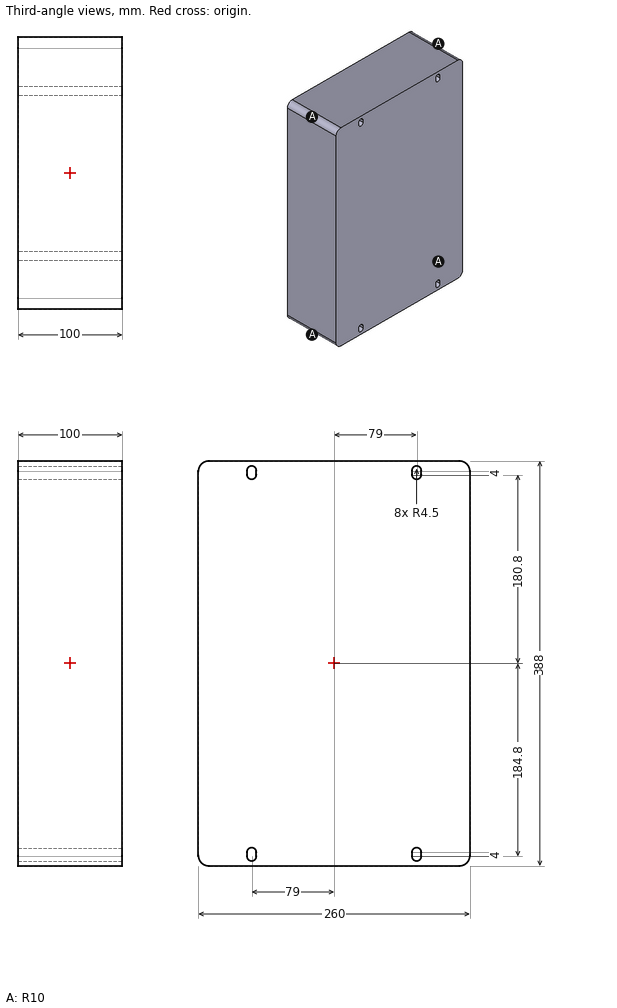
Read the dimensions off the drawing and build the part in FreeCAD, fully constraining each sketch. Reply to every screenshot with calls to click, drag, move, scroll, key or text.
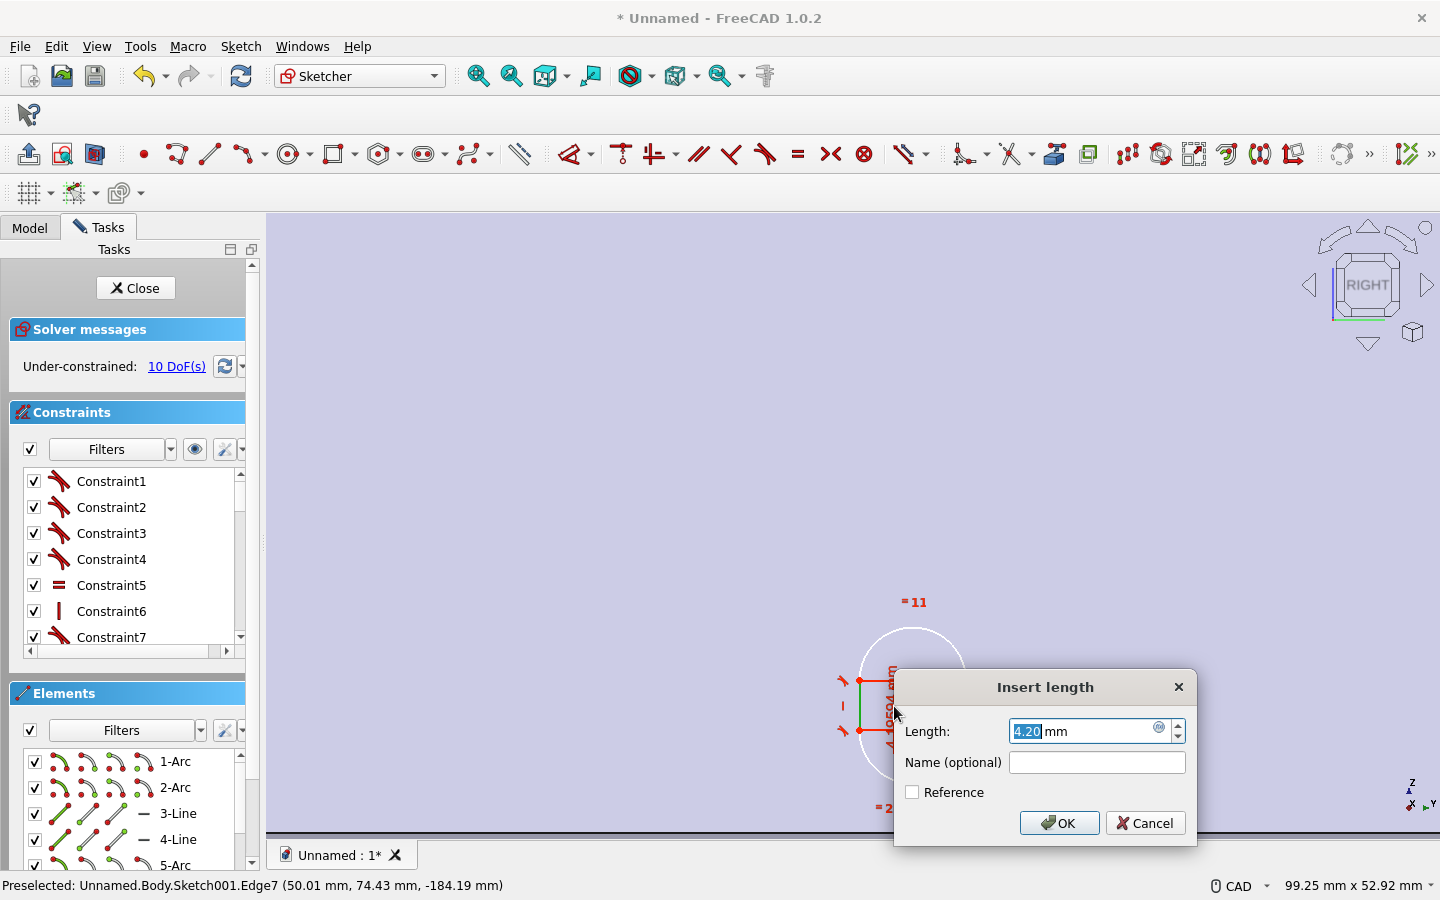
text(4)
key(Return)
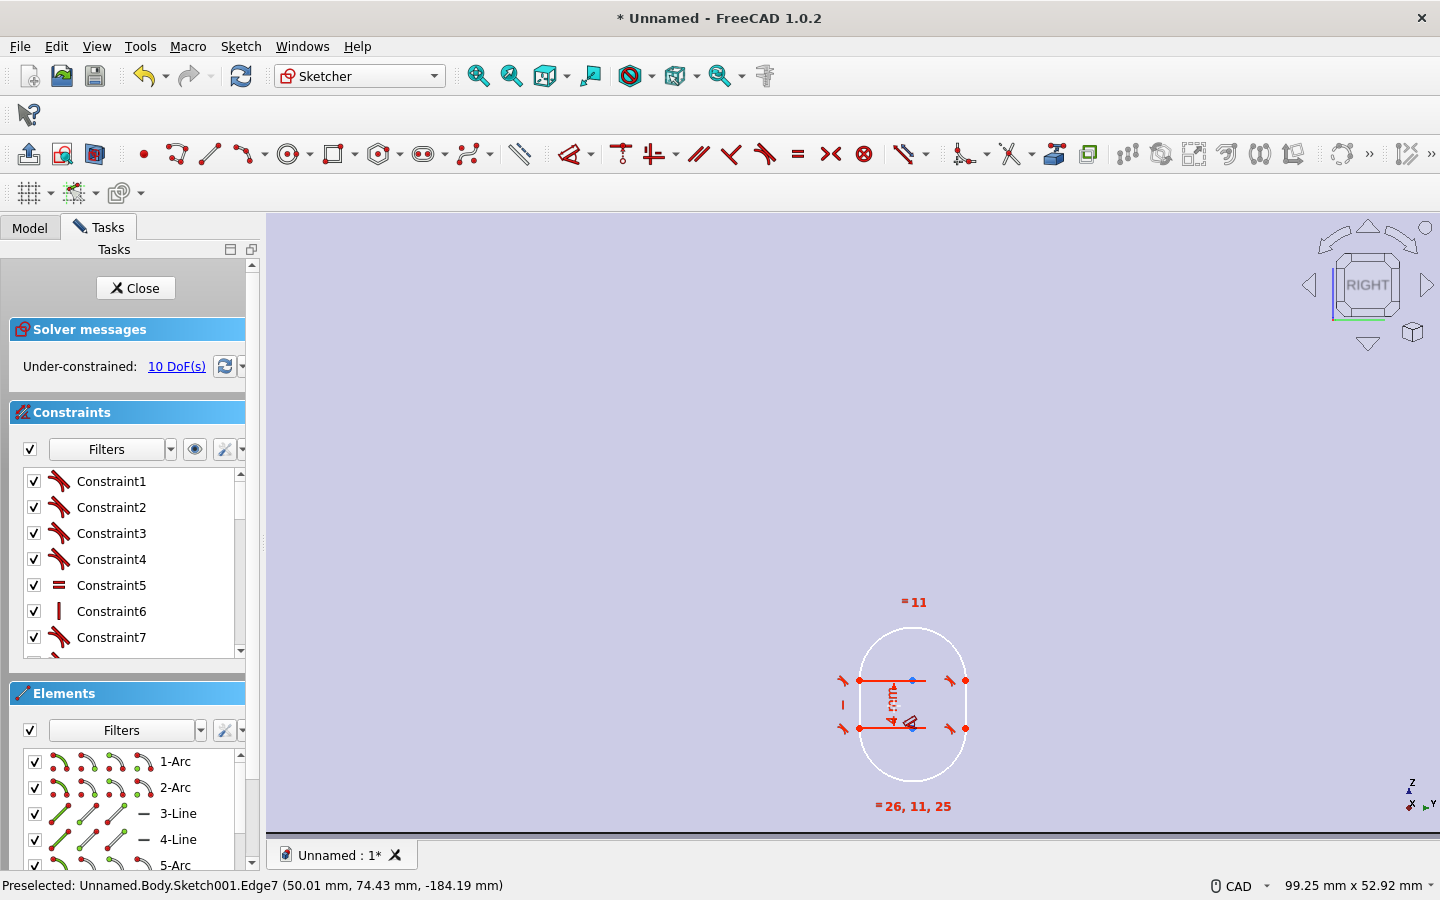
scroll(865, 724, down, 12)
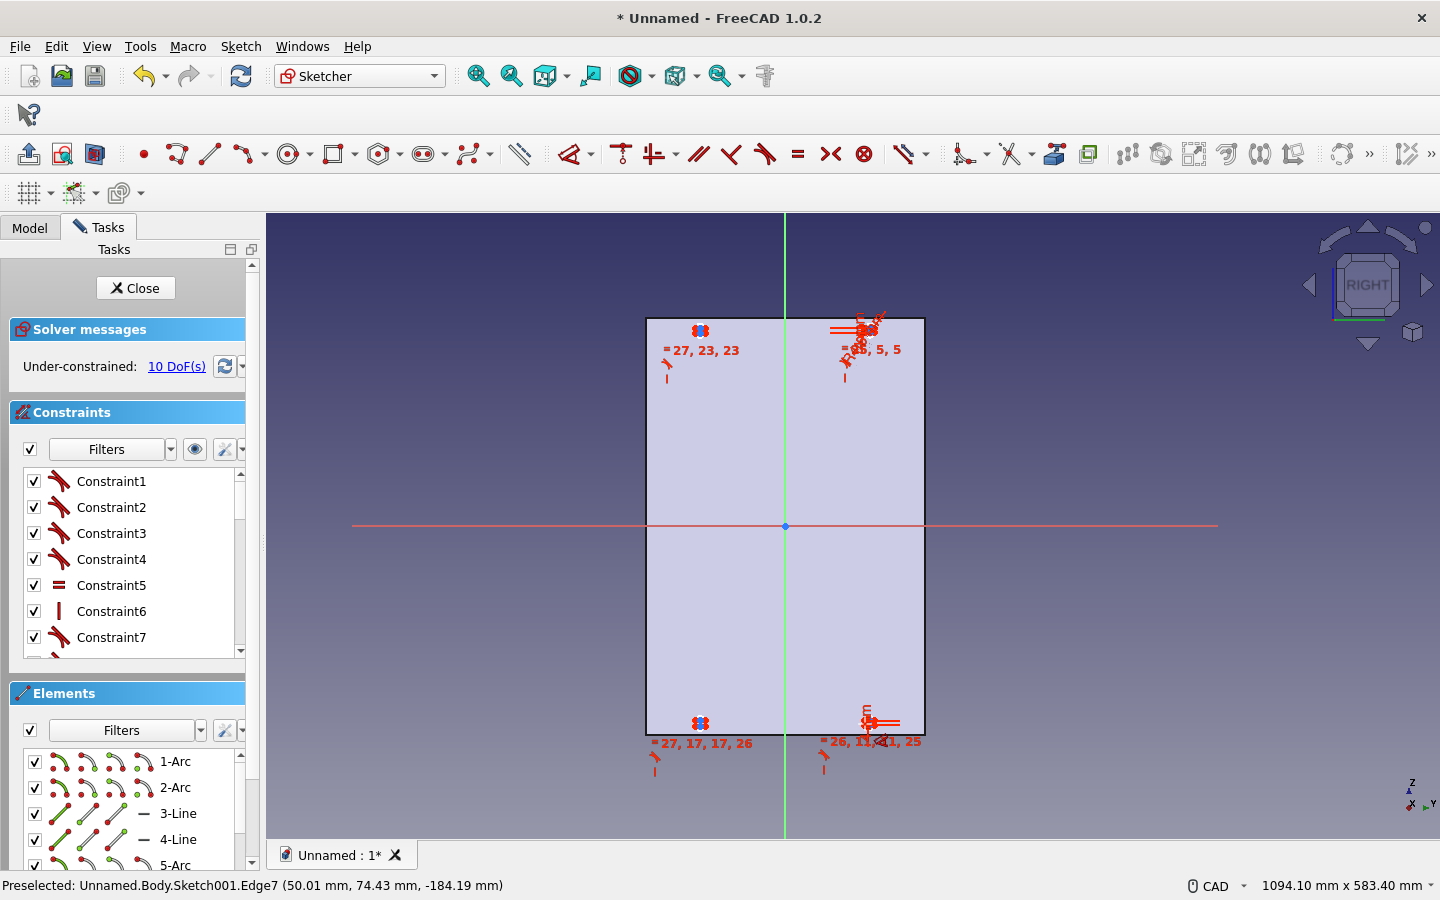
scroll(695, 725, up, 12)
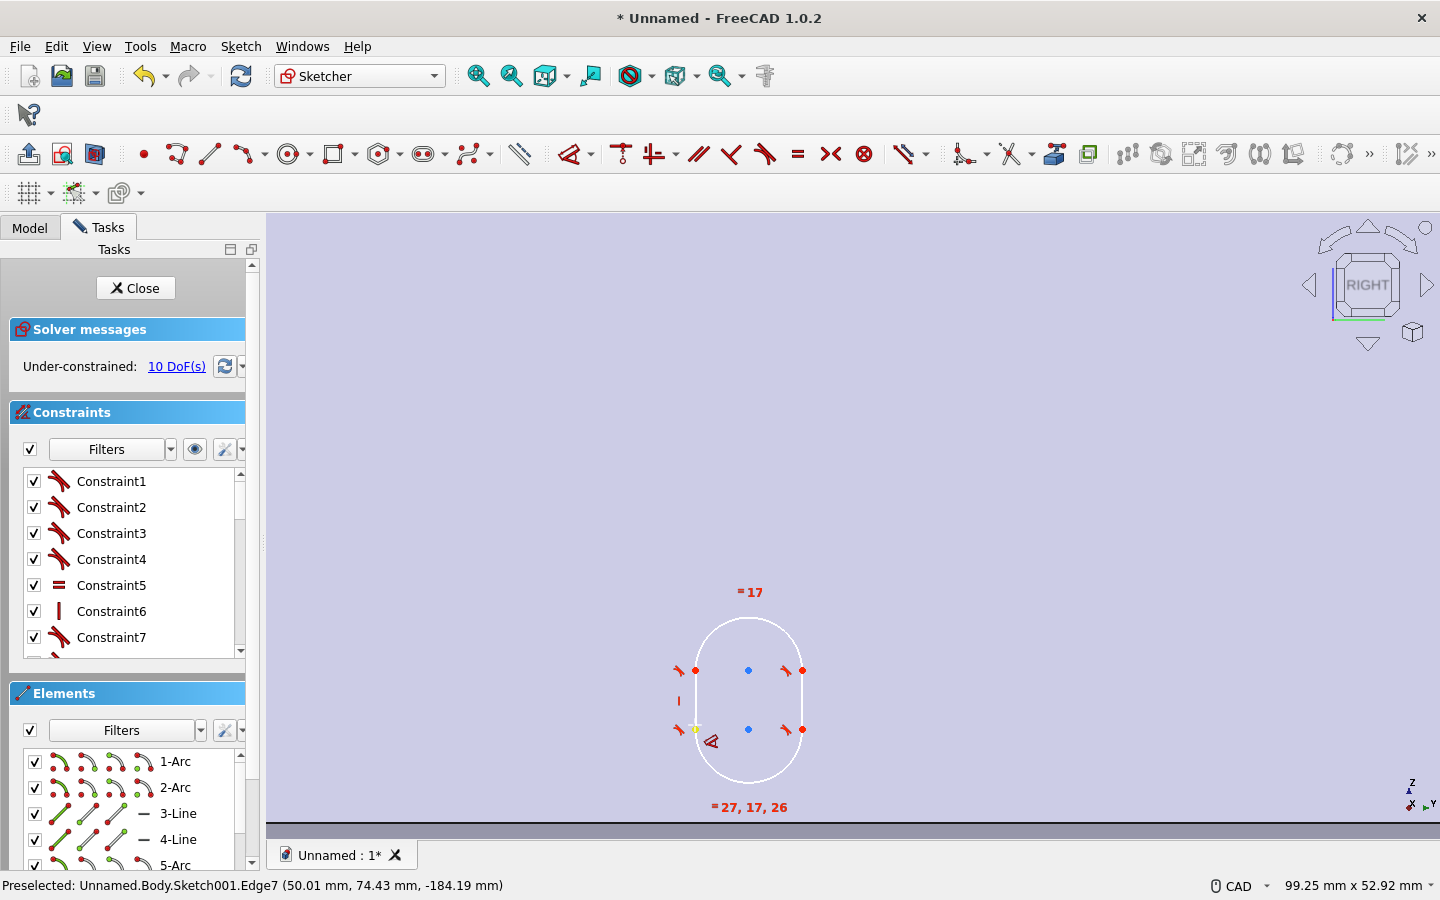
click(696, 712)
click(662, 700)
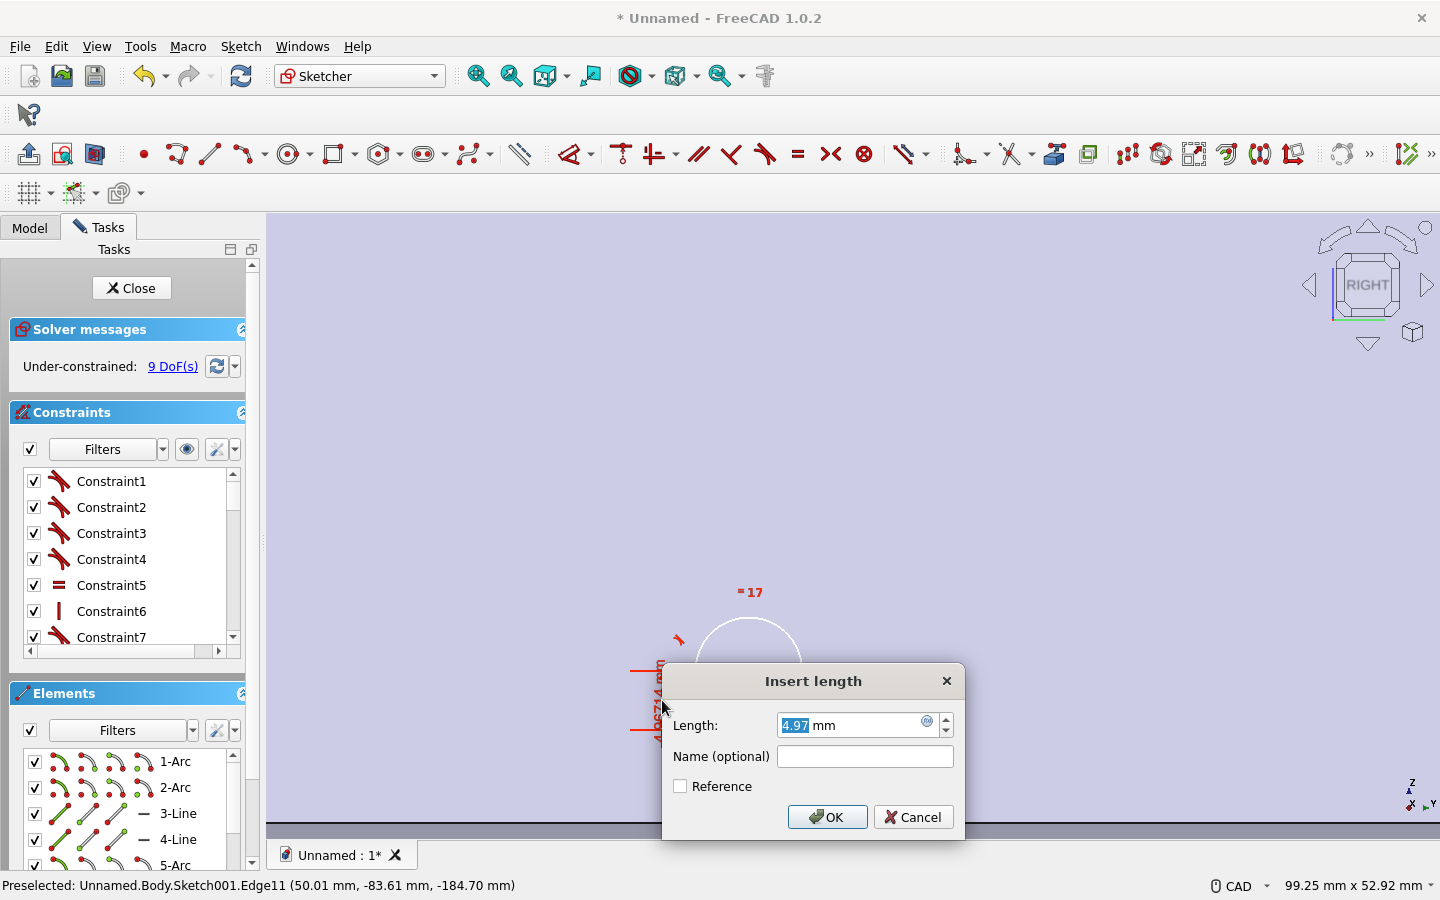
text(4)
key(Return)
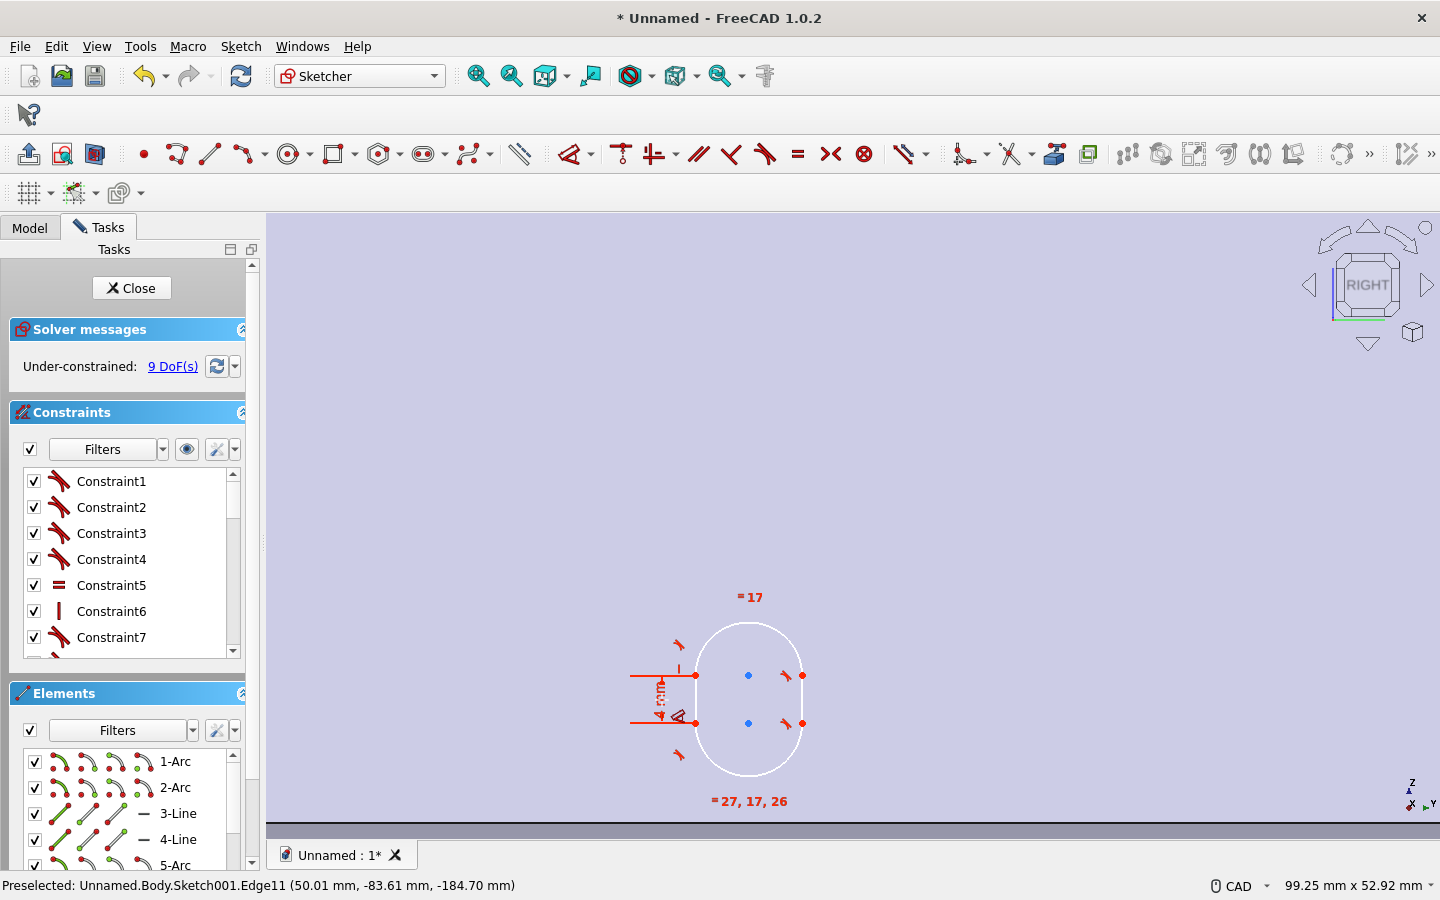
scroll(695, 725, down, 12)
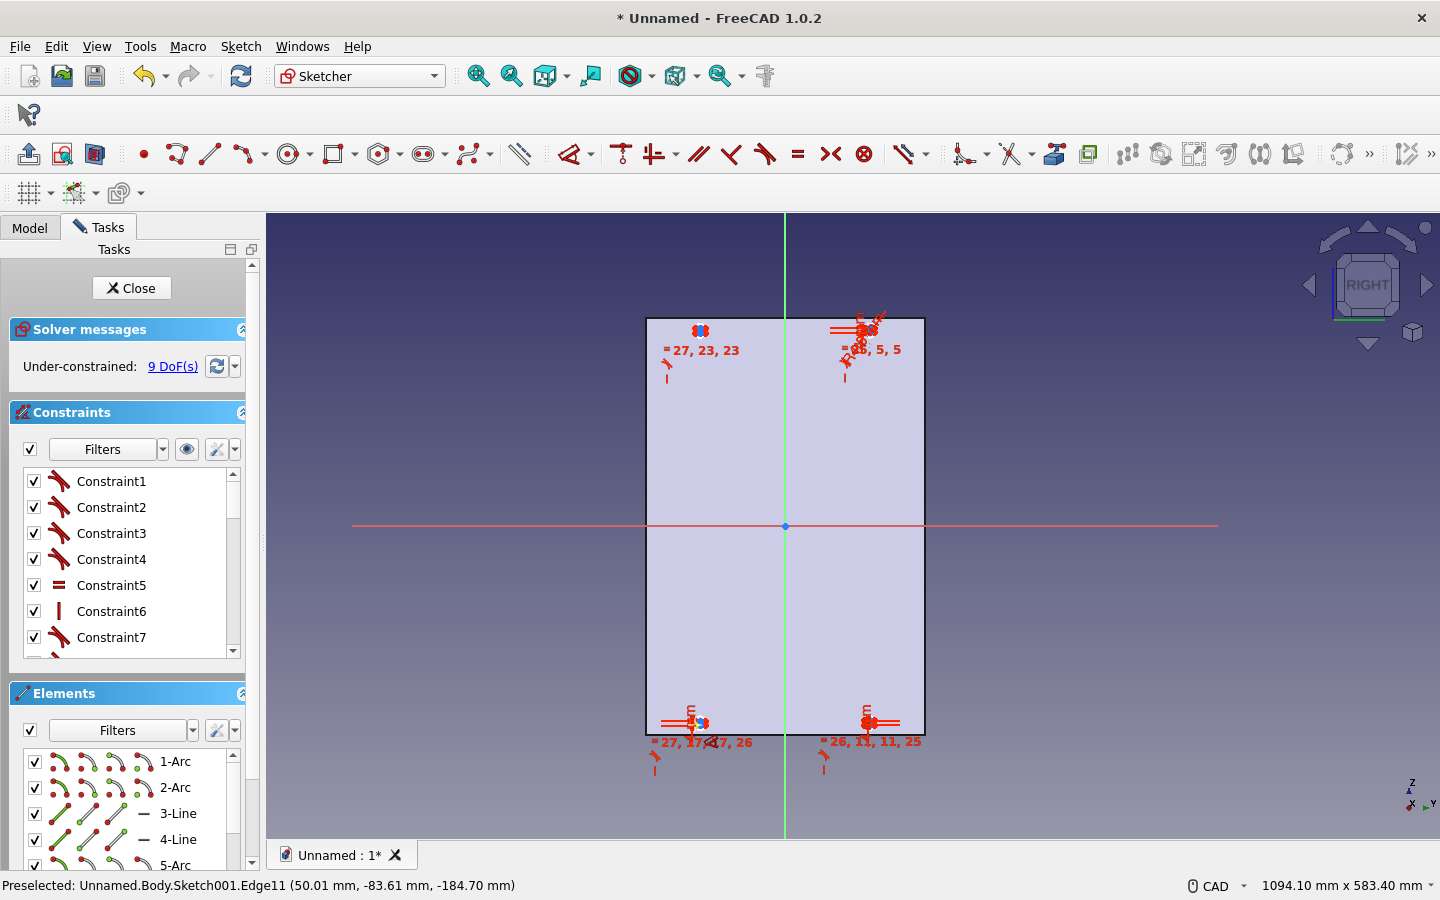
scroll(696, 332, up, 12)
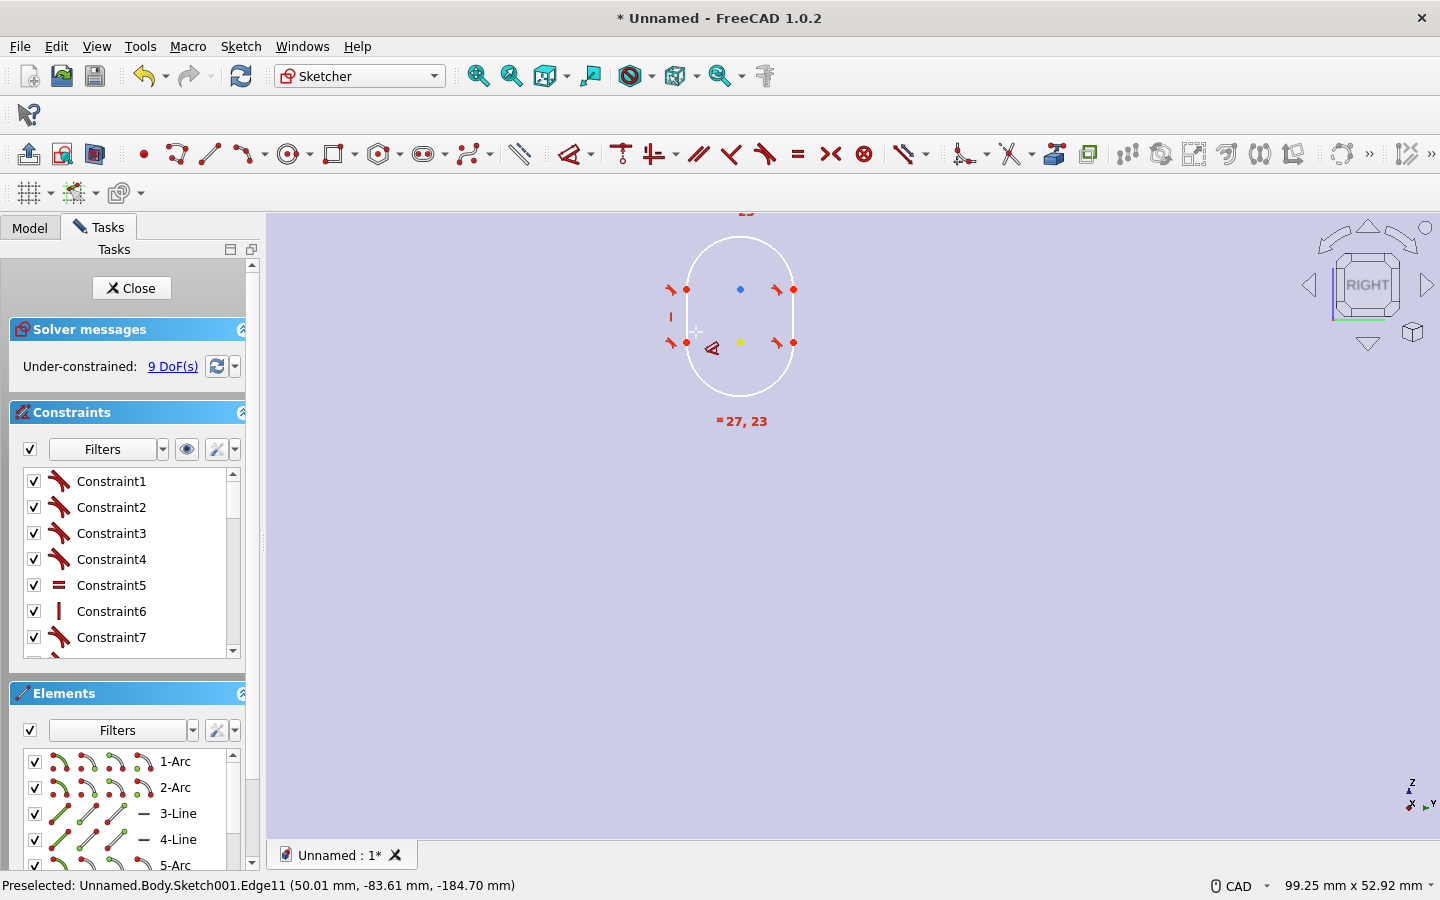
click(687, 327)
click(653, 316)